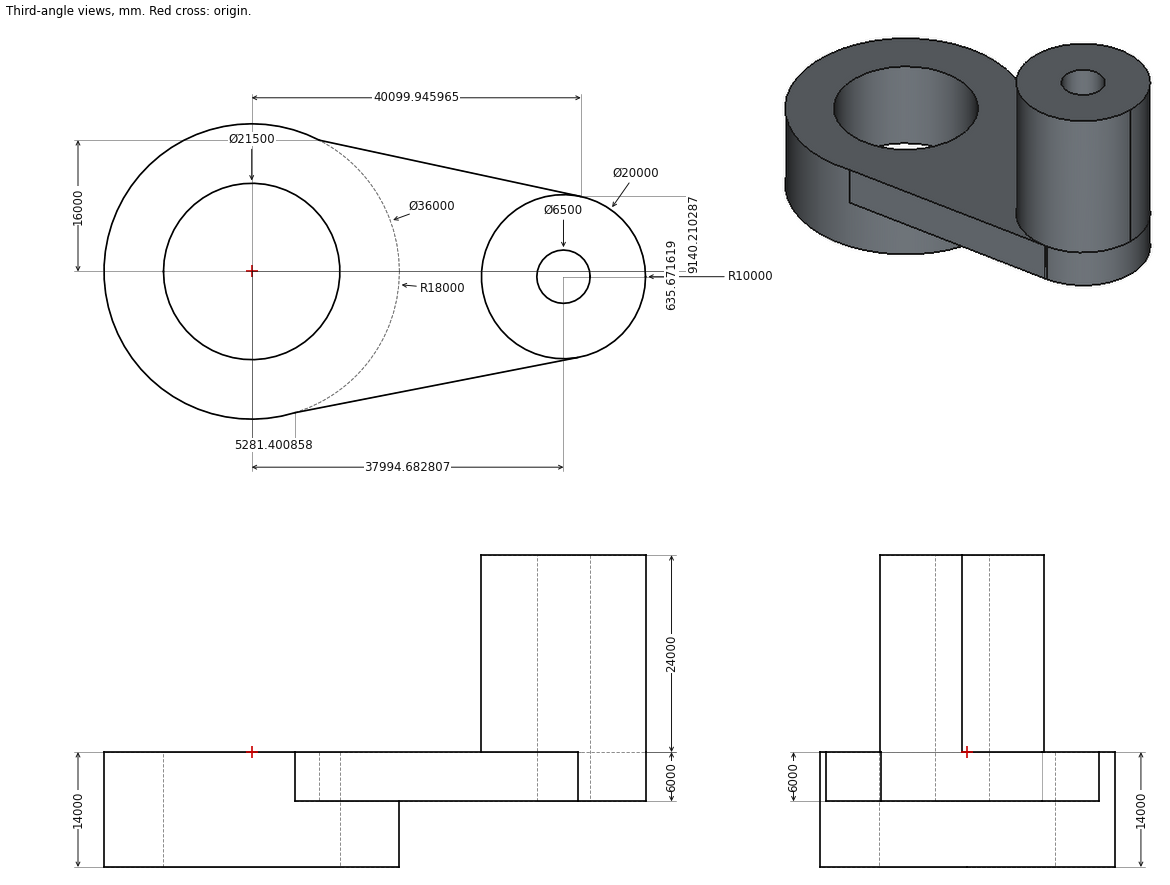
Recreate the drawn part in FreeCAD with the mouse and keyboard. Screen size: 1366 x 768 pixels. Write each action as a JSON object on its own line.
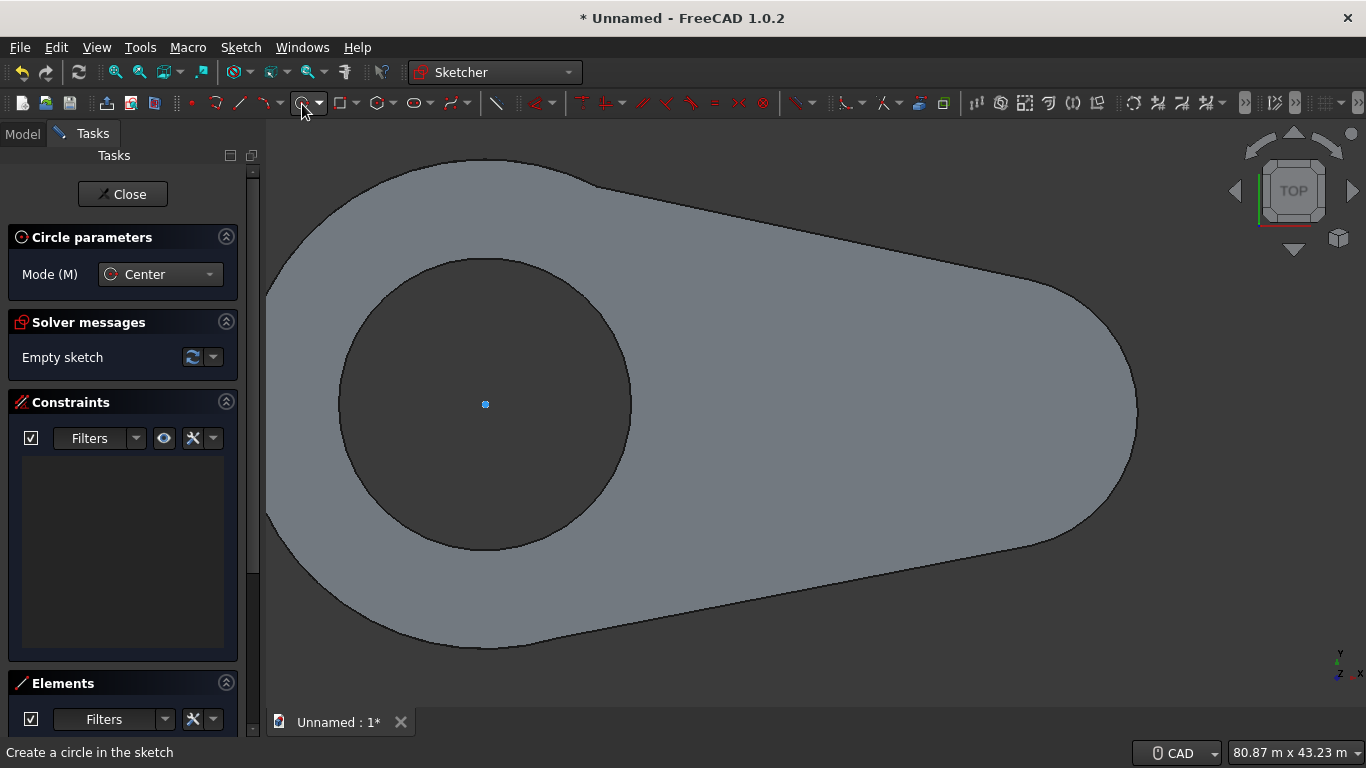
{"action": "scroll", "coordinate": [1002, 413], "scroll_direction": "up", "scroll_amount": 4}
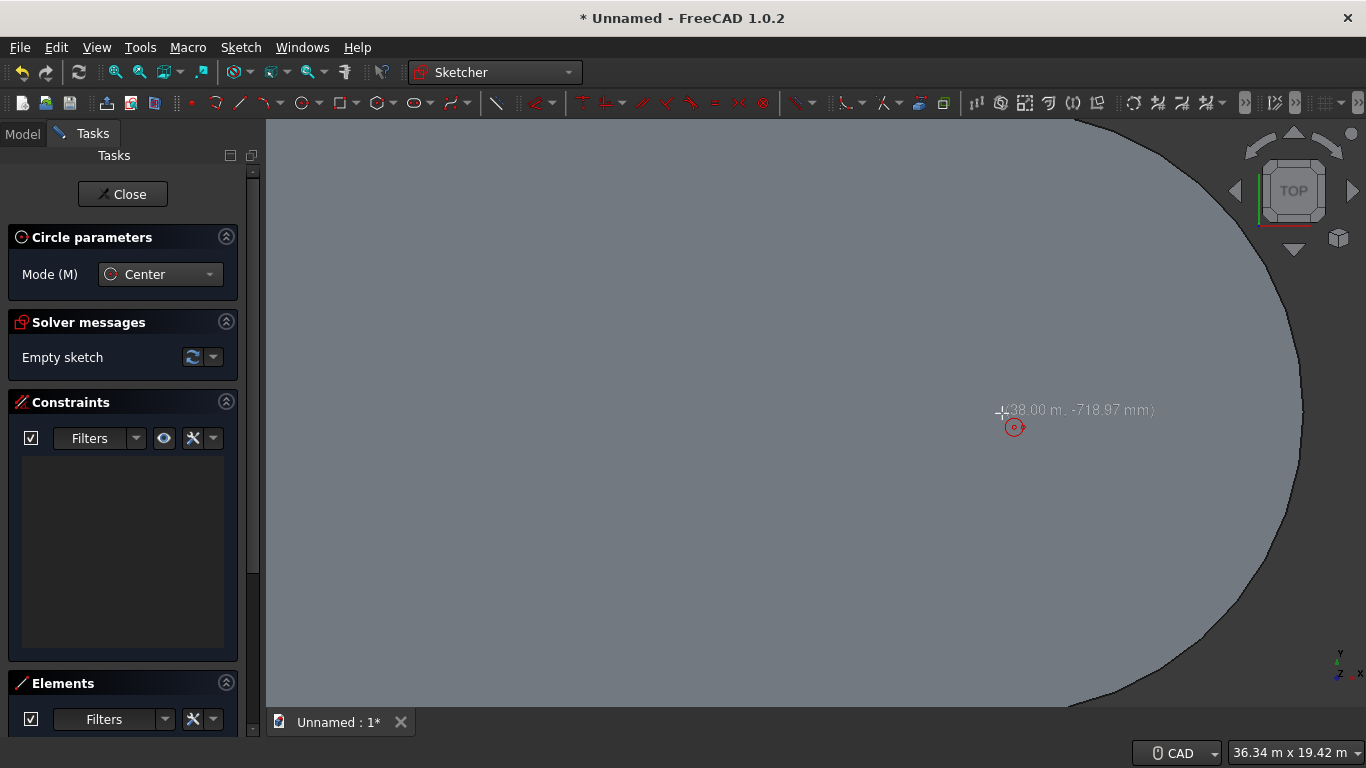
{"action": "left_click", "coordinate": [1001, 412]}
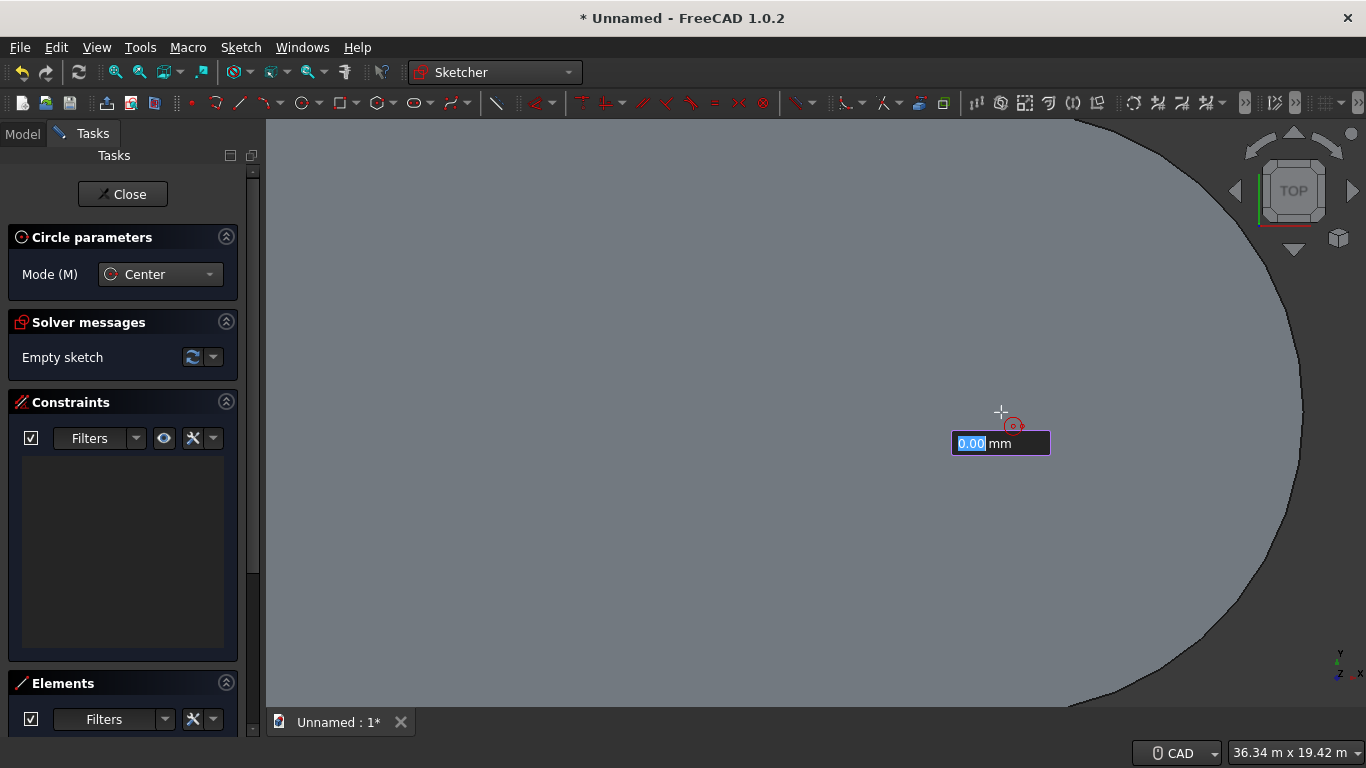
{"action": "scroll", "coordinate": [886, 414], "scroll_direction": "down", "scroll_amount": 4}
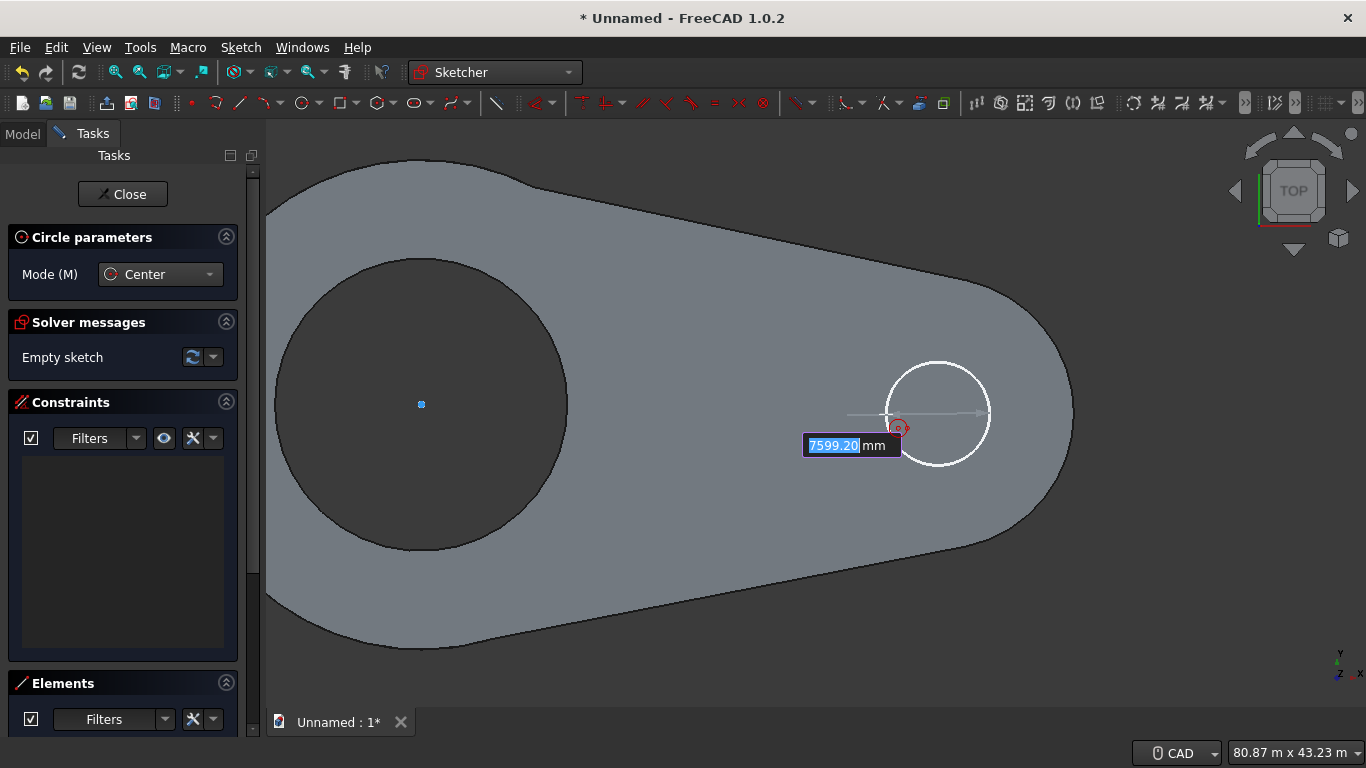
{"action": "left_click", "coordinate": [1034, 317]}
{"action": "key", "text": "Escape"}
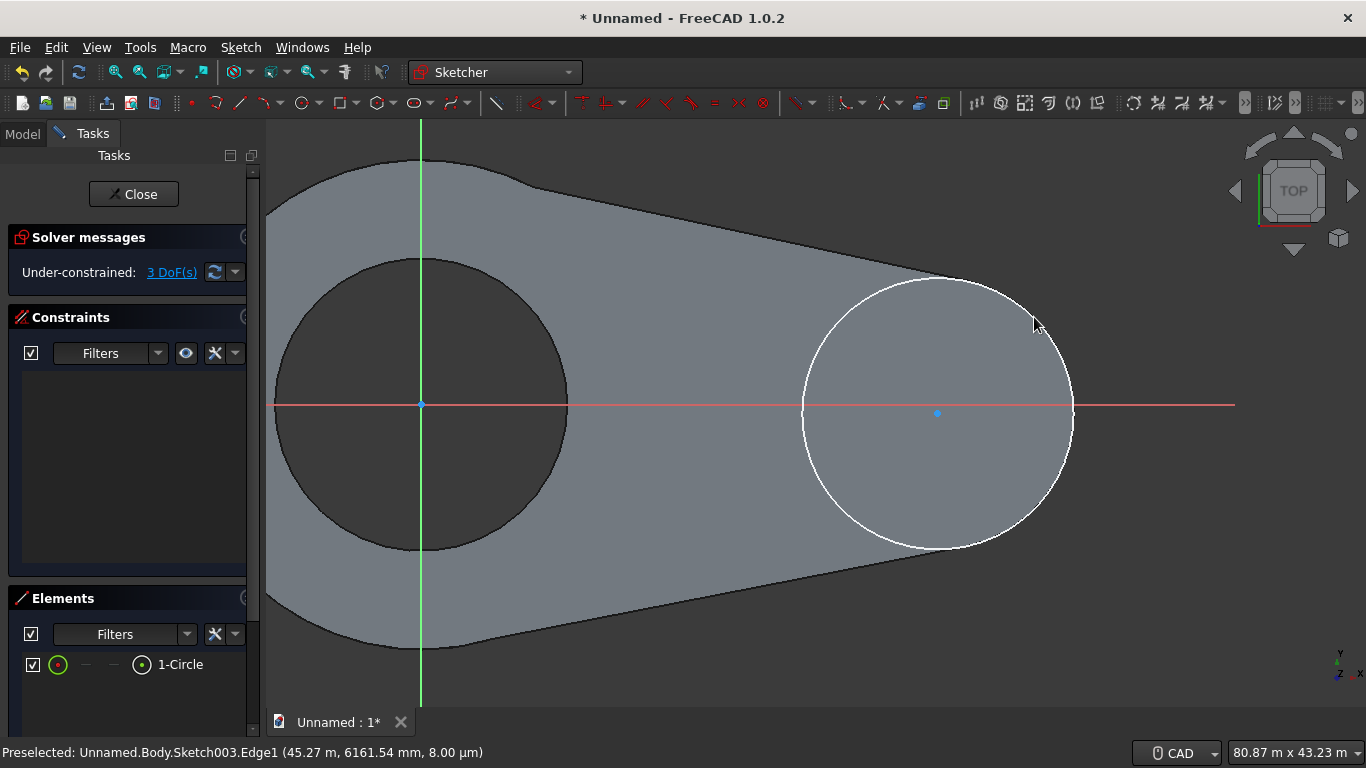
{"action": "left_click", "coordinate": [536, 104]}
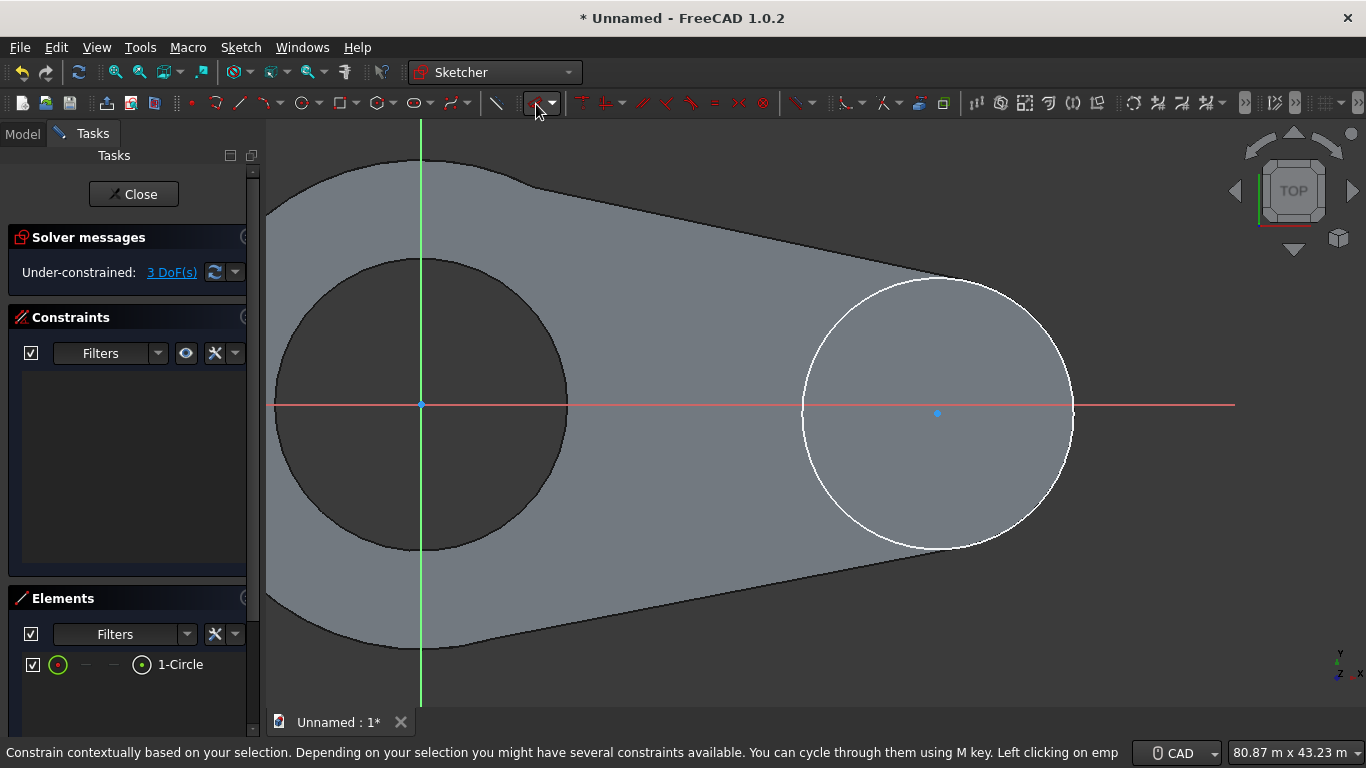
{"action": "left_click", "coordinate": [1034, 318]}
{"action": "left_click", "coordinate": [1057, 295]}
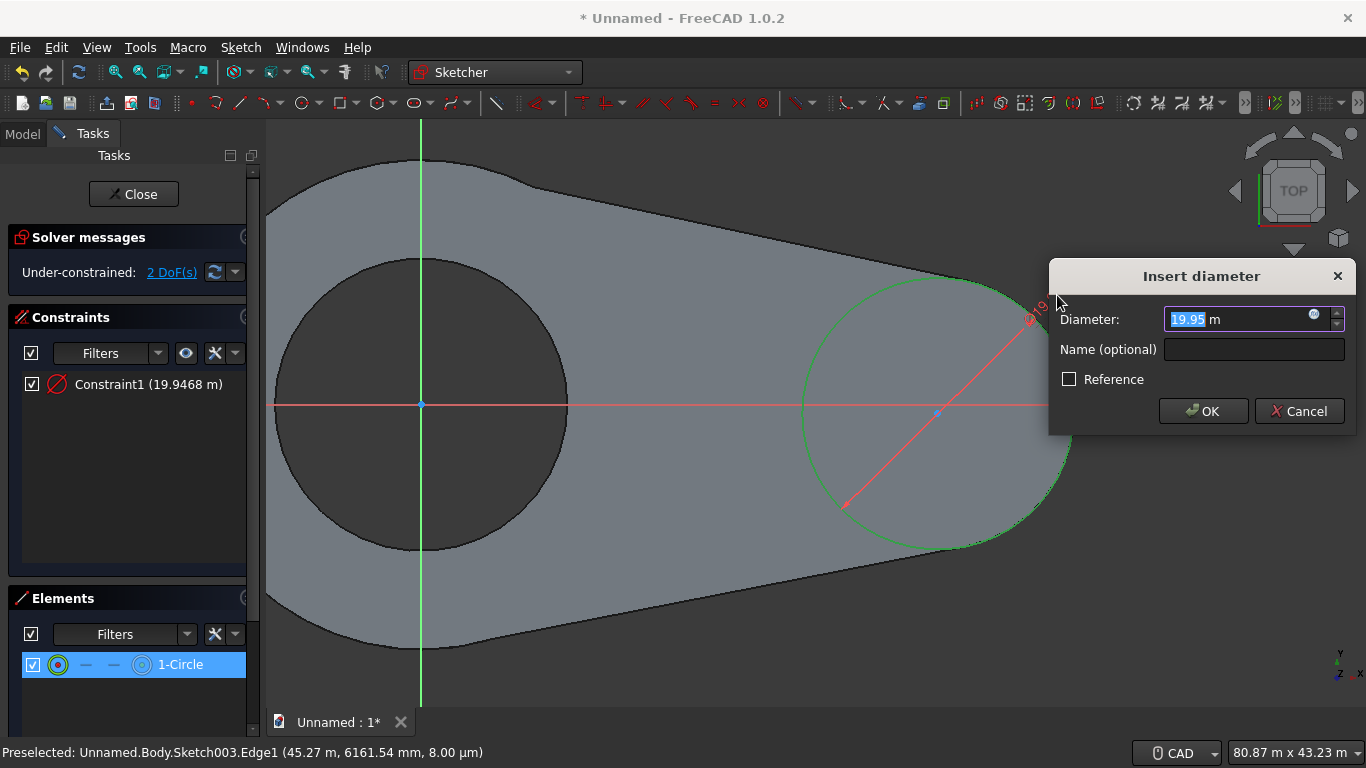
{"action": "key", "text": "ctrl+a"}
{"action": "type", "text": "20000 mm"}
{"action": "key", "text": "Return"}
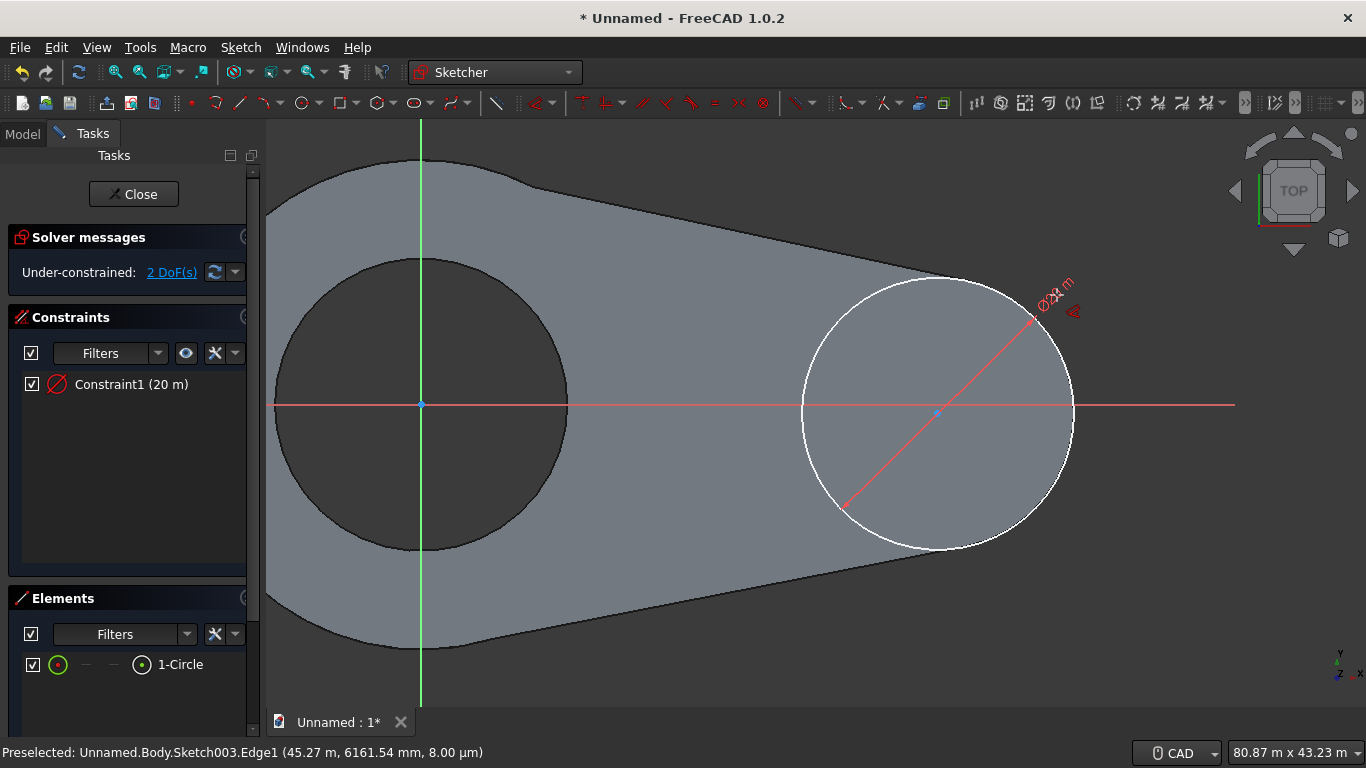
{"action": "scroll", "coordinate": [938, 414], "scroll_direction": "up", "scroll_amount": 8}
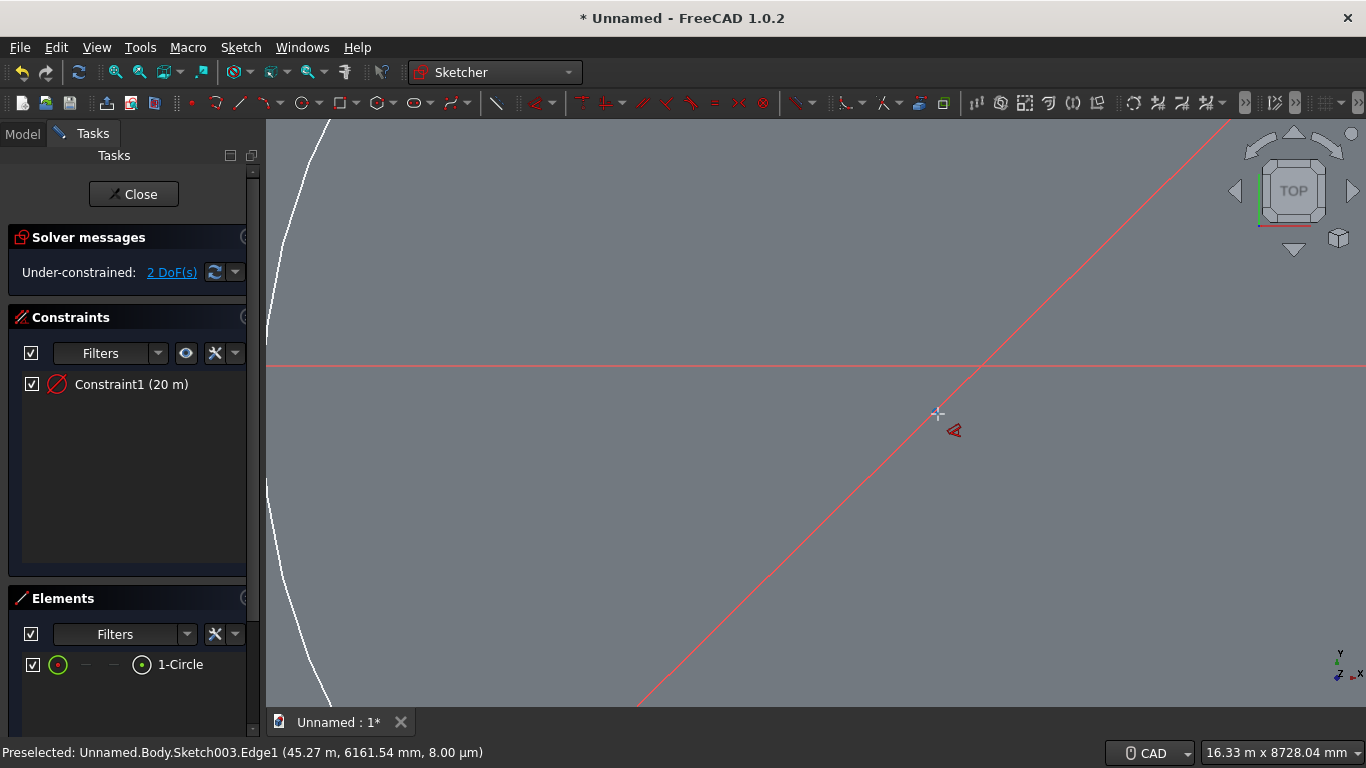
{"action": "left_click", "coordinate": [936, 411]}
{"action": "left_click", "coordinate": [970, 389]}